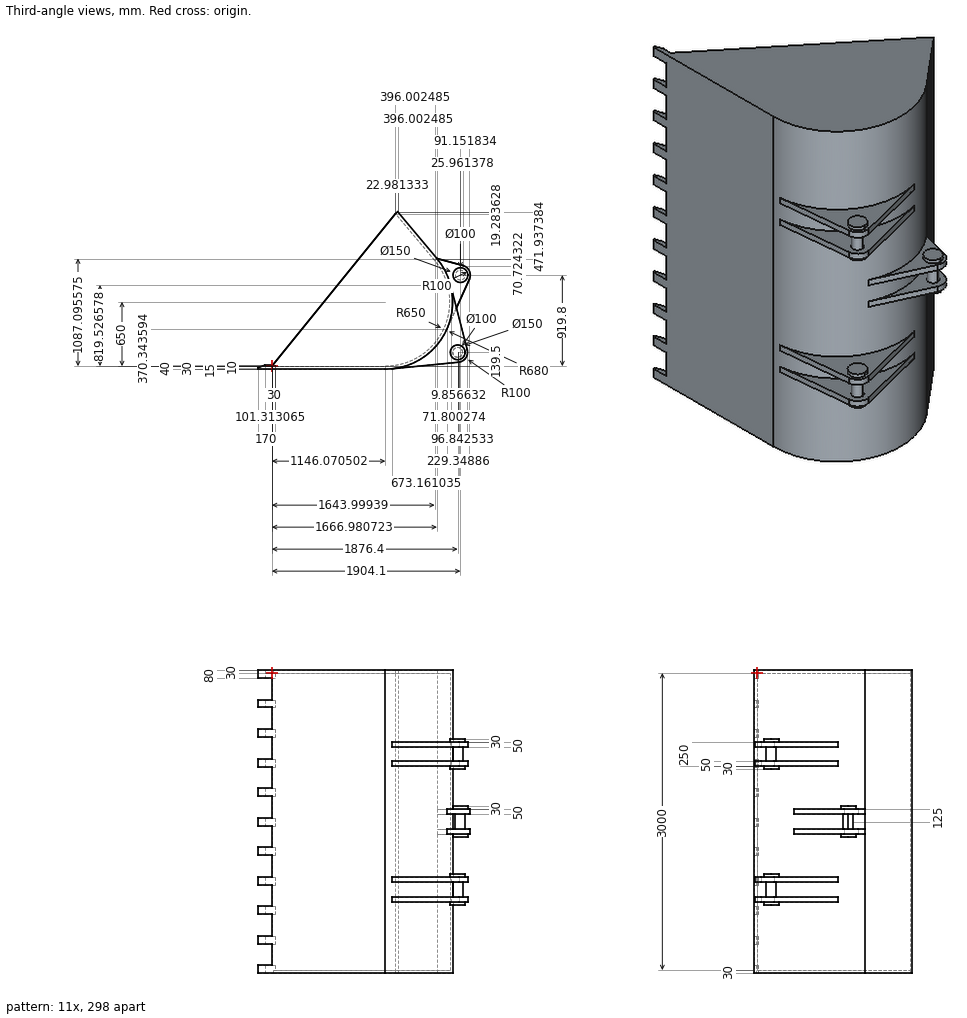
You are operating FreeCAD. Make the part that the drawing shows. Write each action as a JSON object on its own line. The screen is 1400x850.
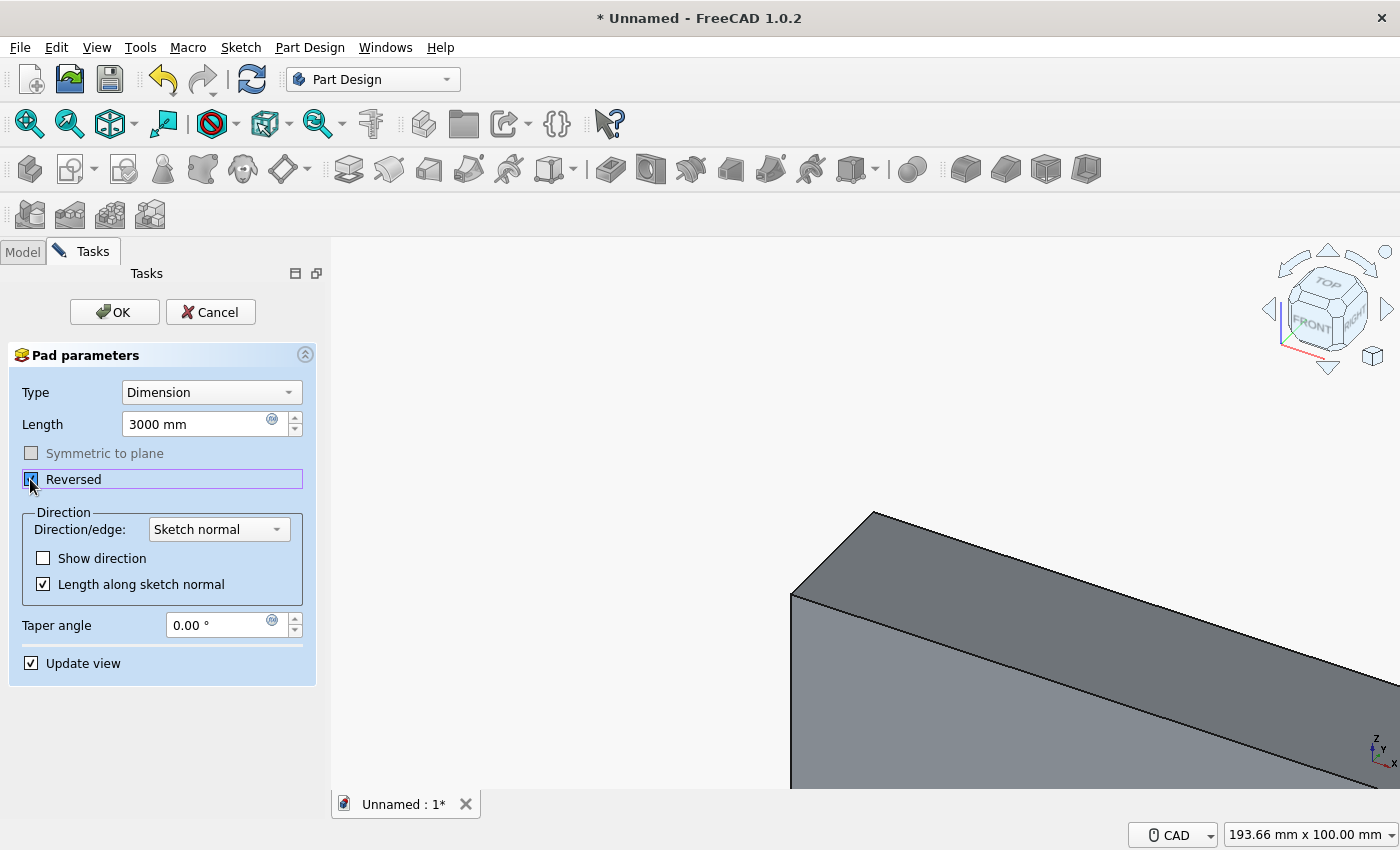
{"action": "left_click", "coordinate": [115, 312]}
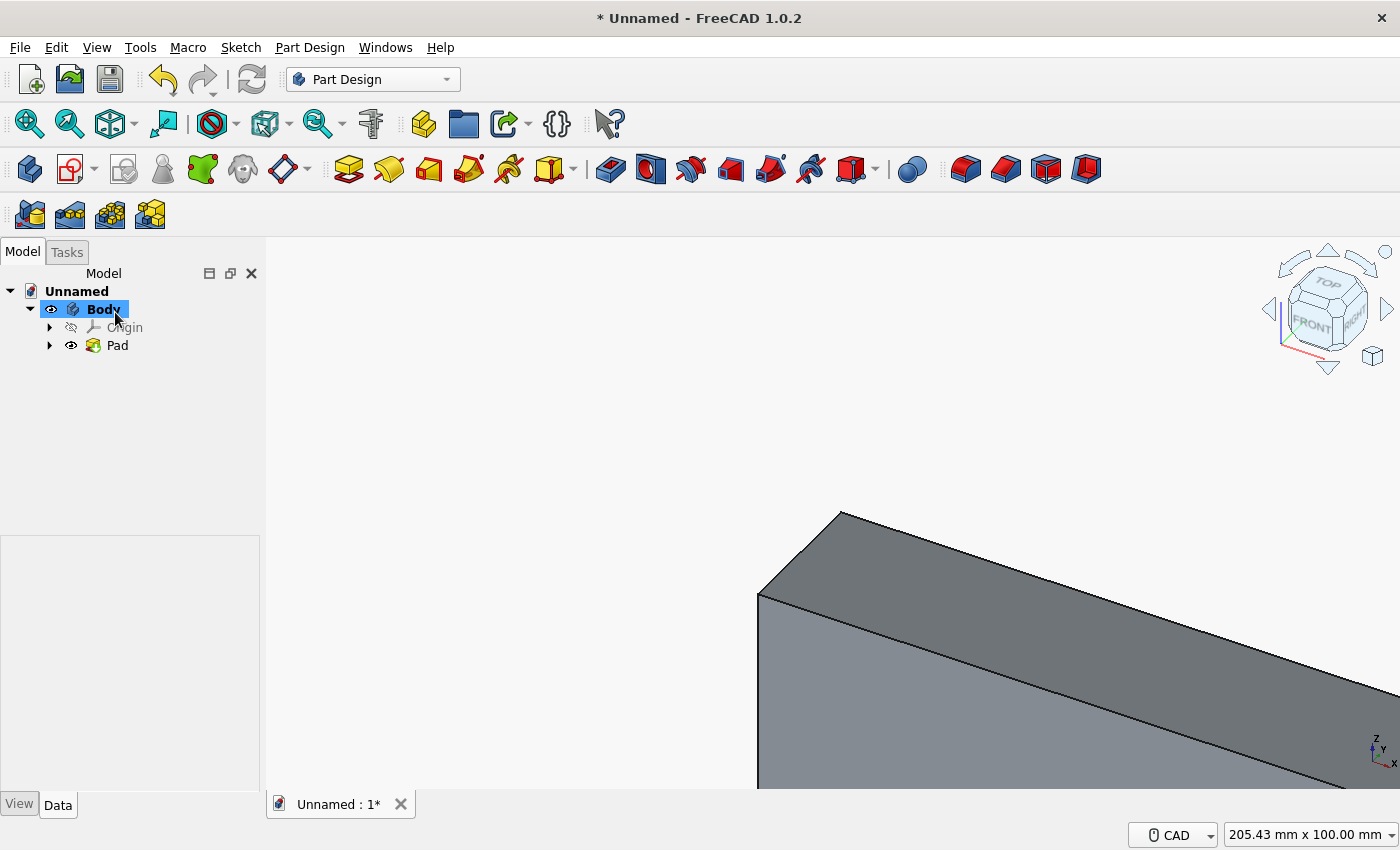
{"action": "left_click", "coordinate": [30, 124]}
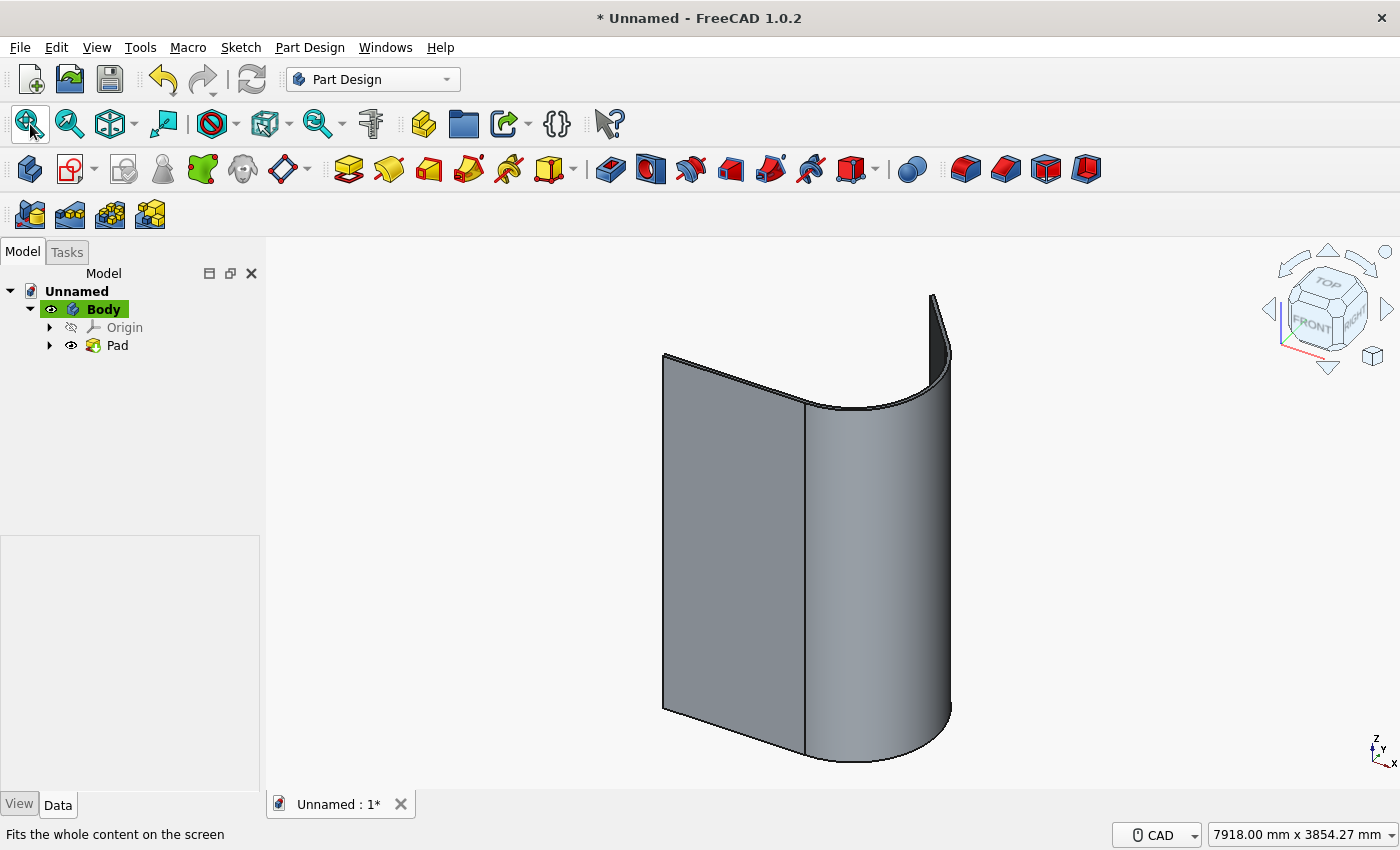
{"action": "left_click", "coordinate": [50, 327]}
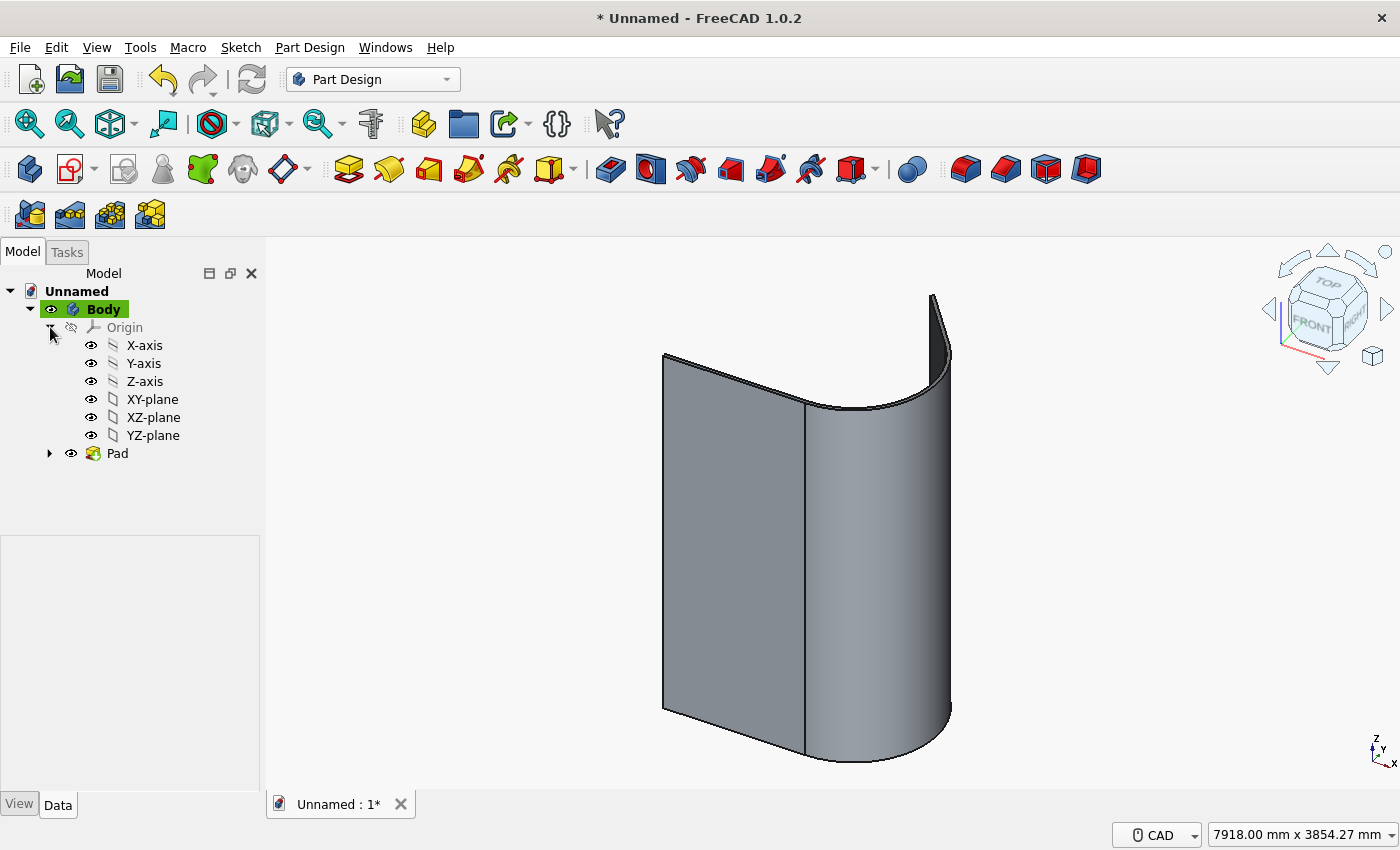
{"action": "left_click", "coordinate": [136, 399]}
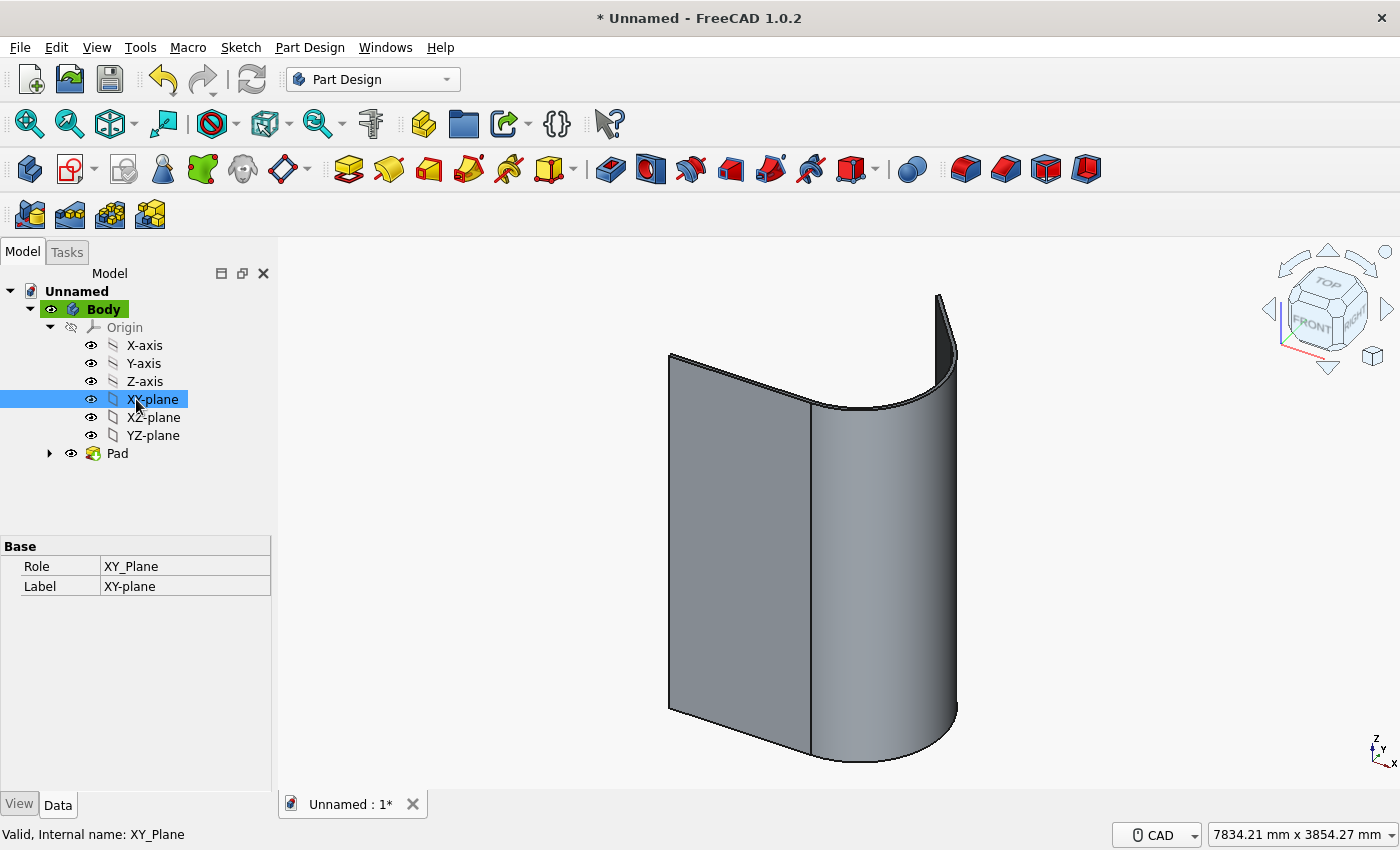
{"action": "left_click", "coordinate": [284, 170]}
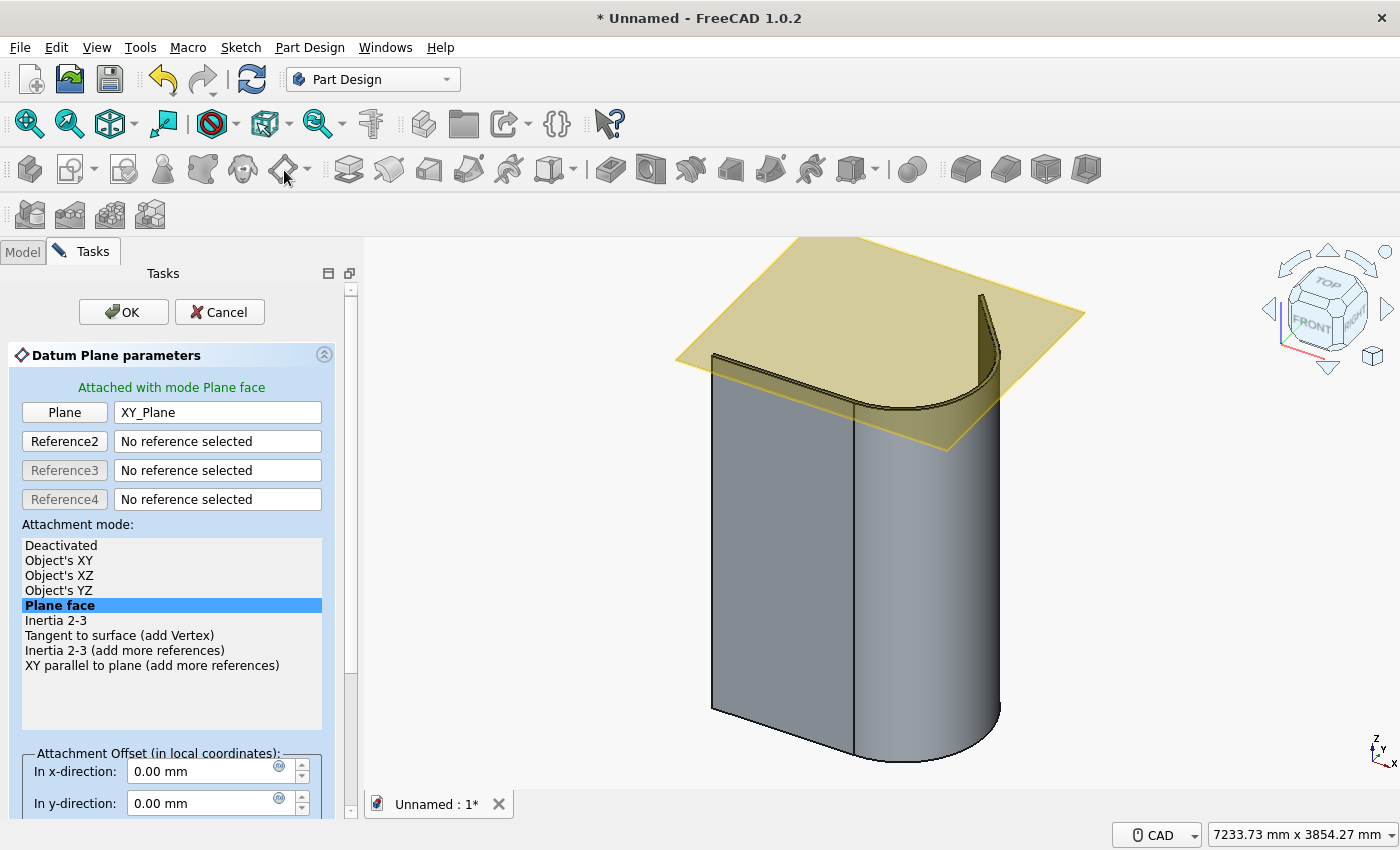
{"action": "scroll", "coordinate": [351, 550], "scroll_direction": "down", "scroll_amount": 2}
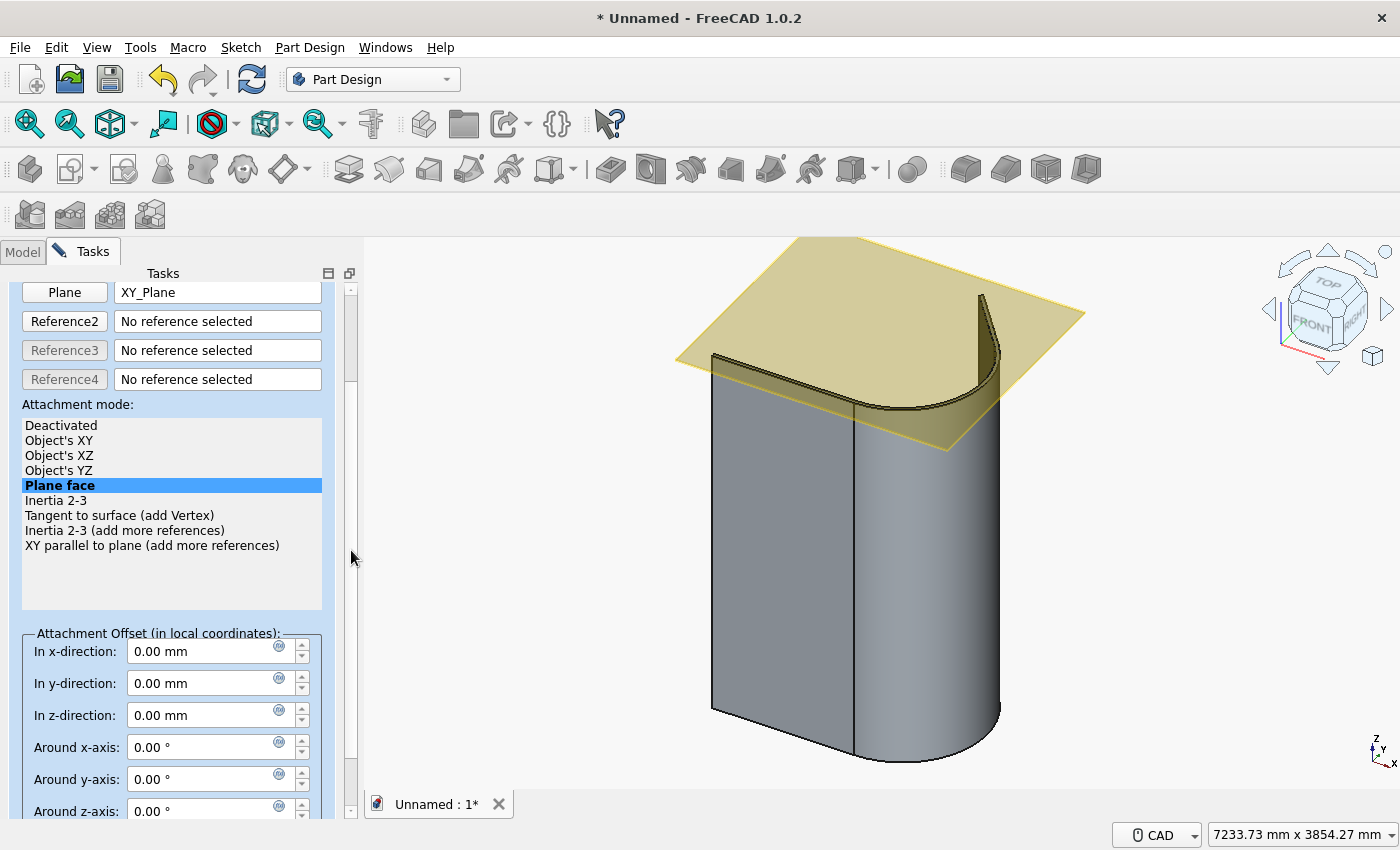
{"action": "triple_click", "coordinate": [210, 715]}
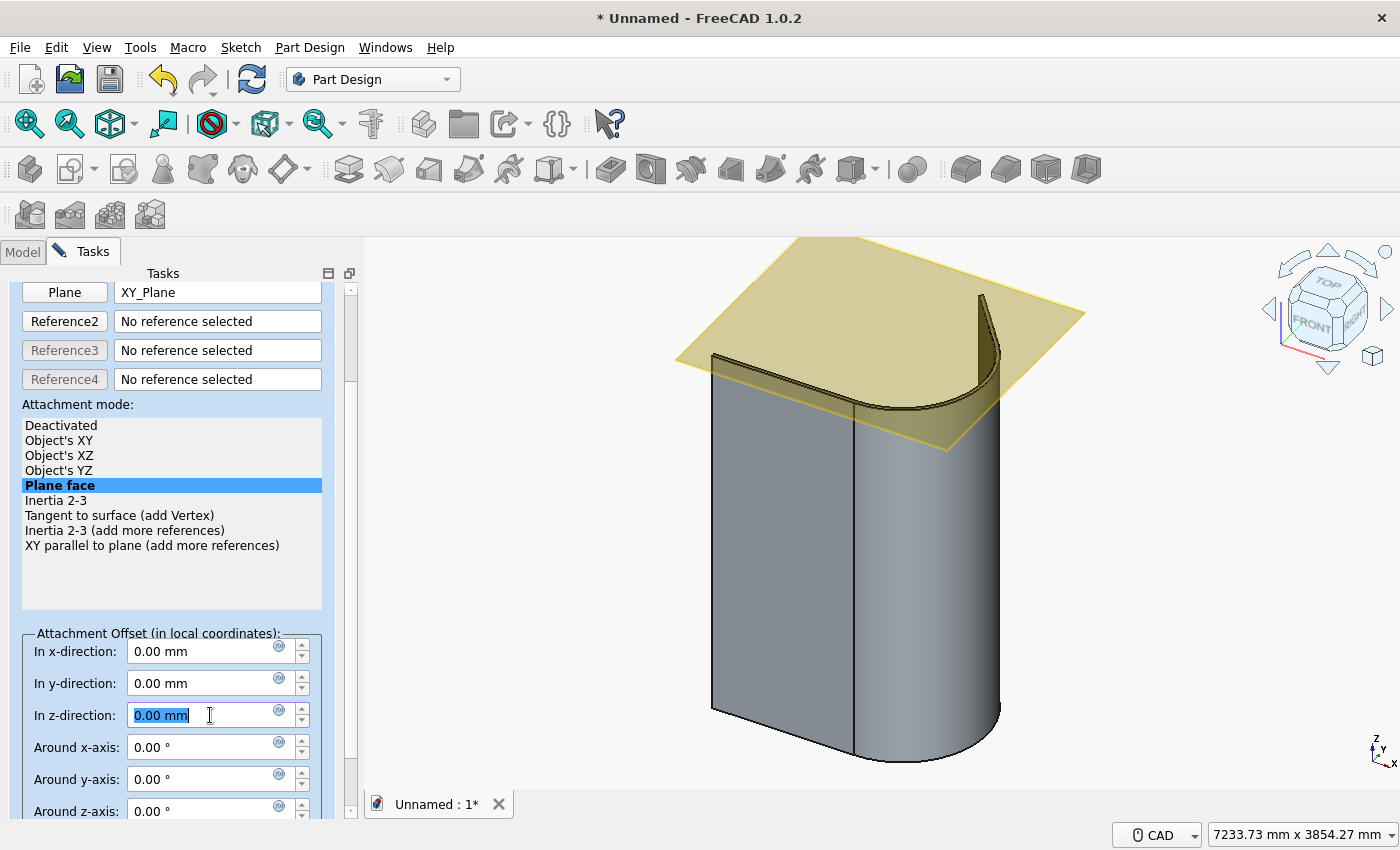
{"action": "type", "text": "30"}
{"action": "key", "text": "Tab"}